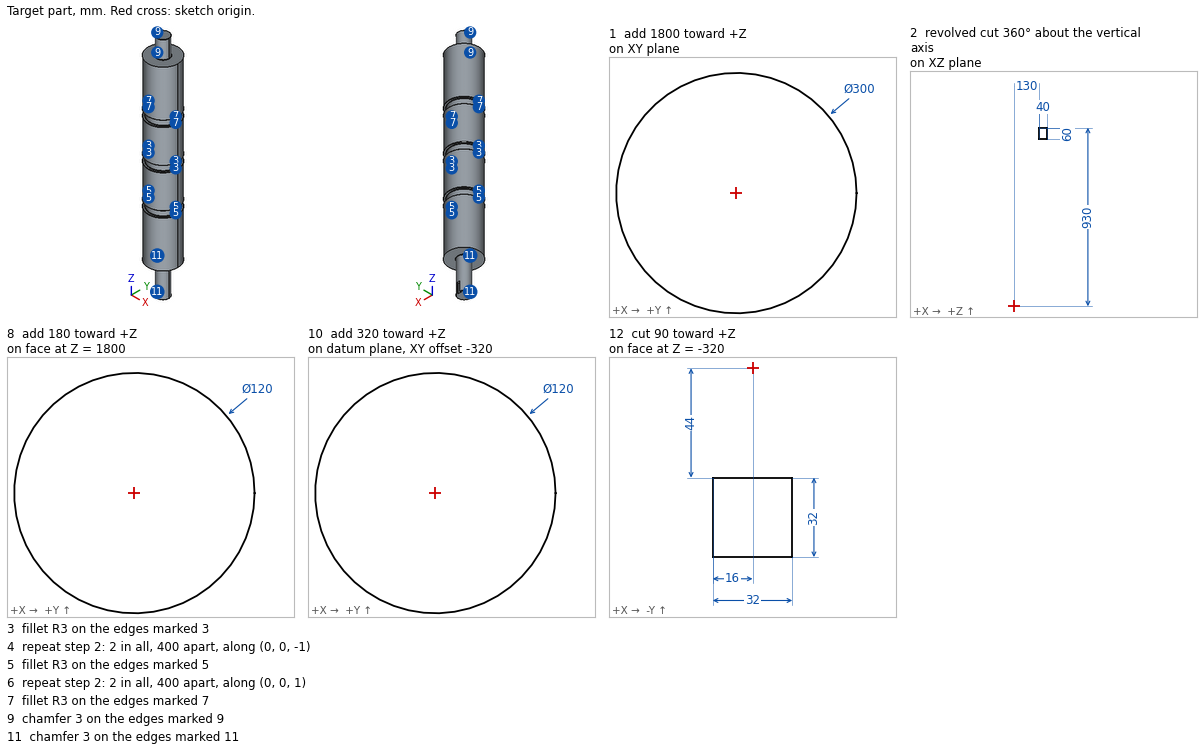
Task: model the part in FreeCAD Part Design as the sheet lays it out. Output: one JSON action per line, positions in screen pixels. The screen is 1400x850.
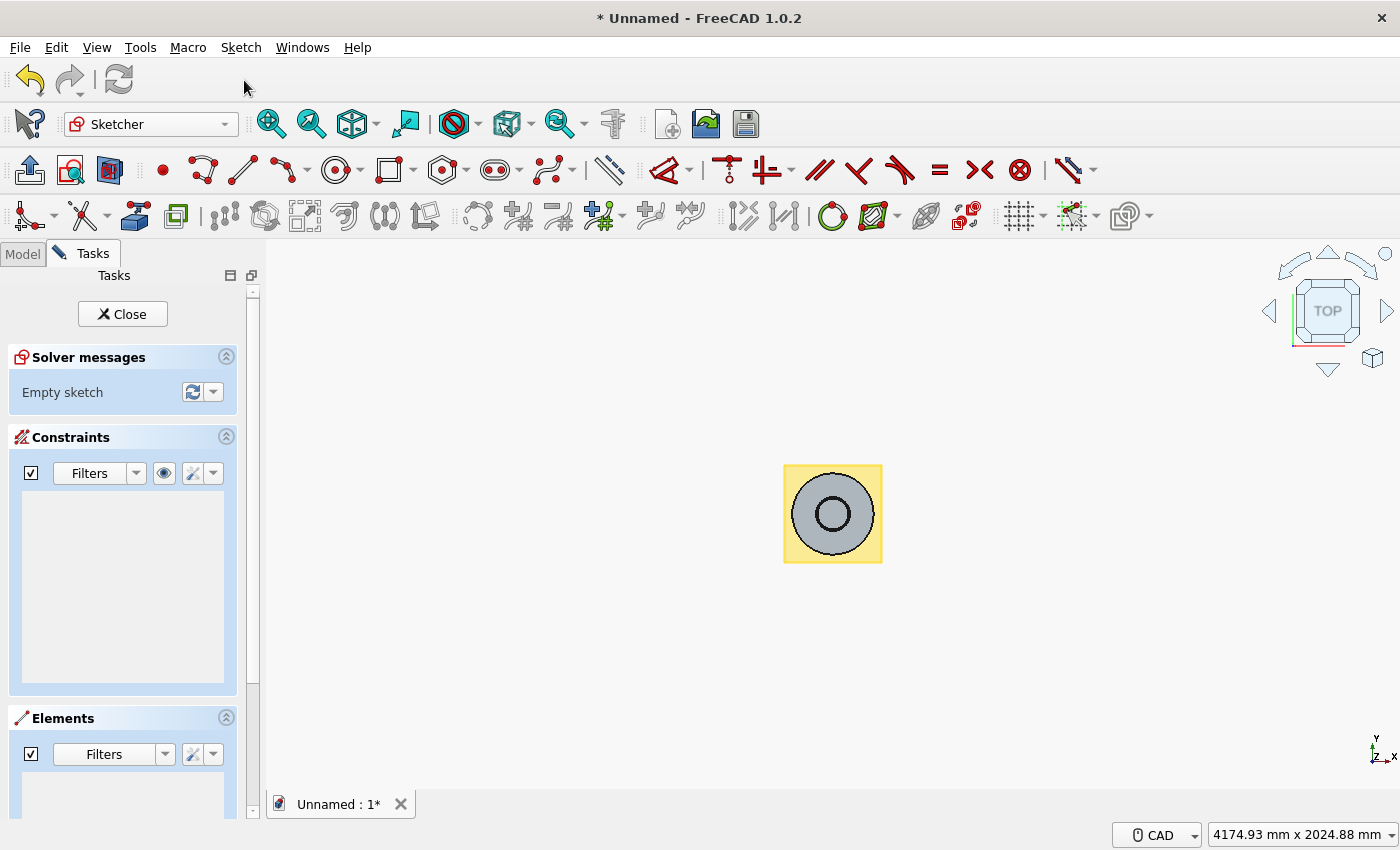
{"action": "left_click", "coordinate": [110, 170]}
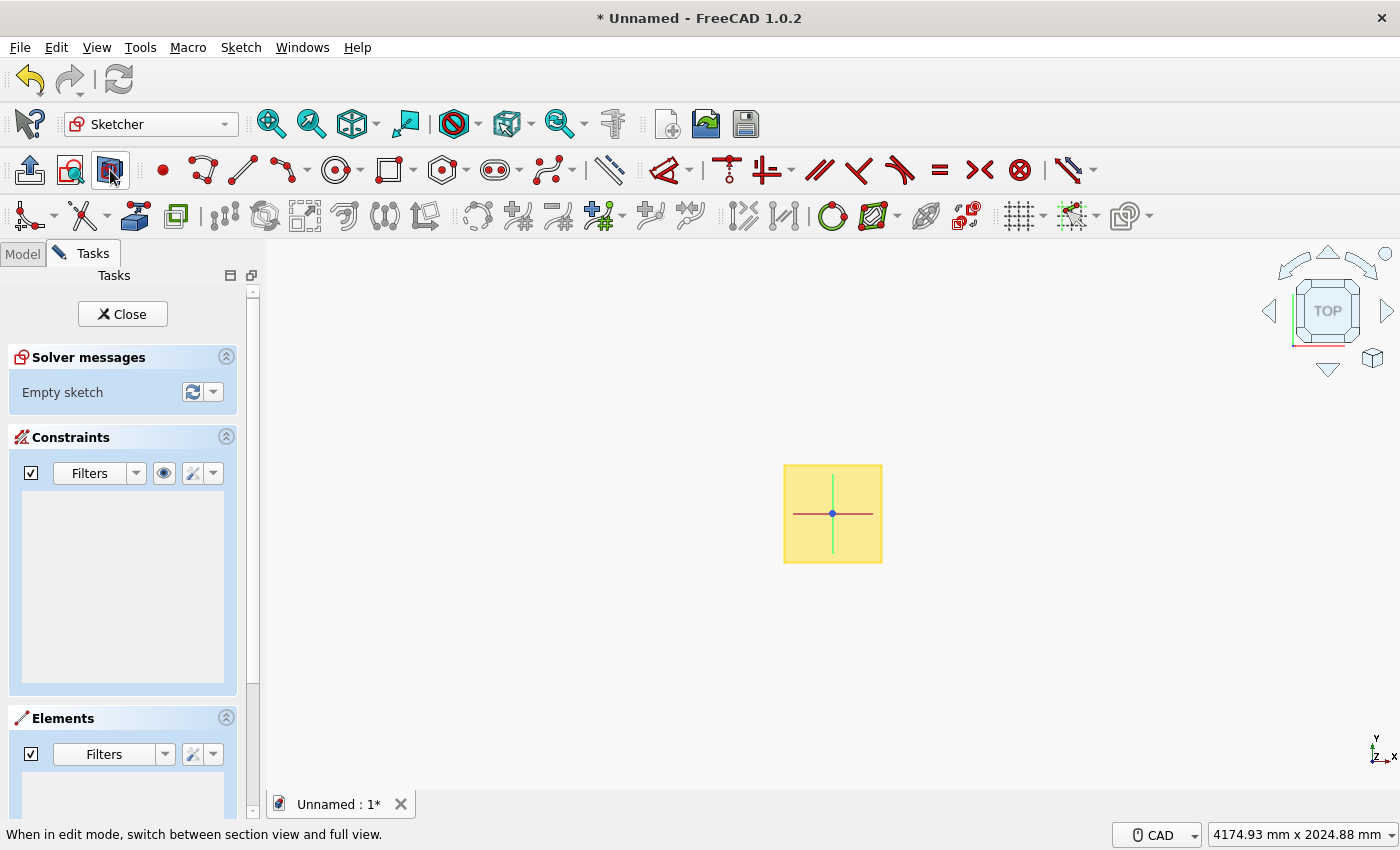
{"action": "scroll", "coordinate": [840, 514], "scroll_direction": "up", "scroll_amount": 12}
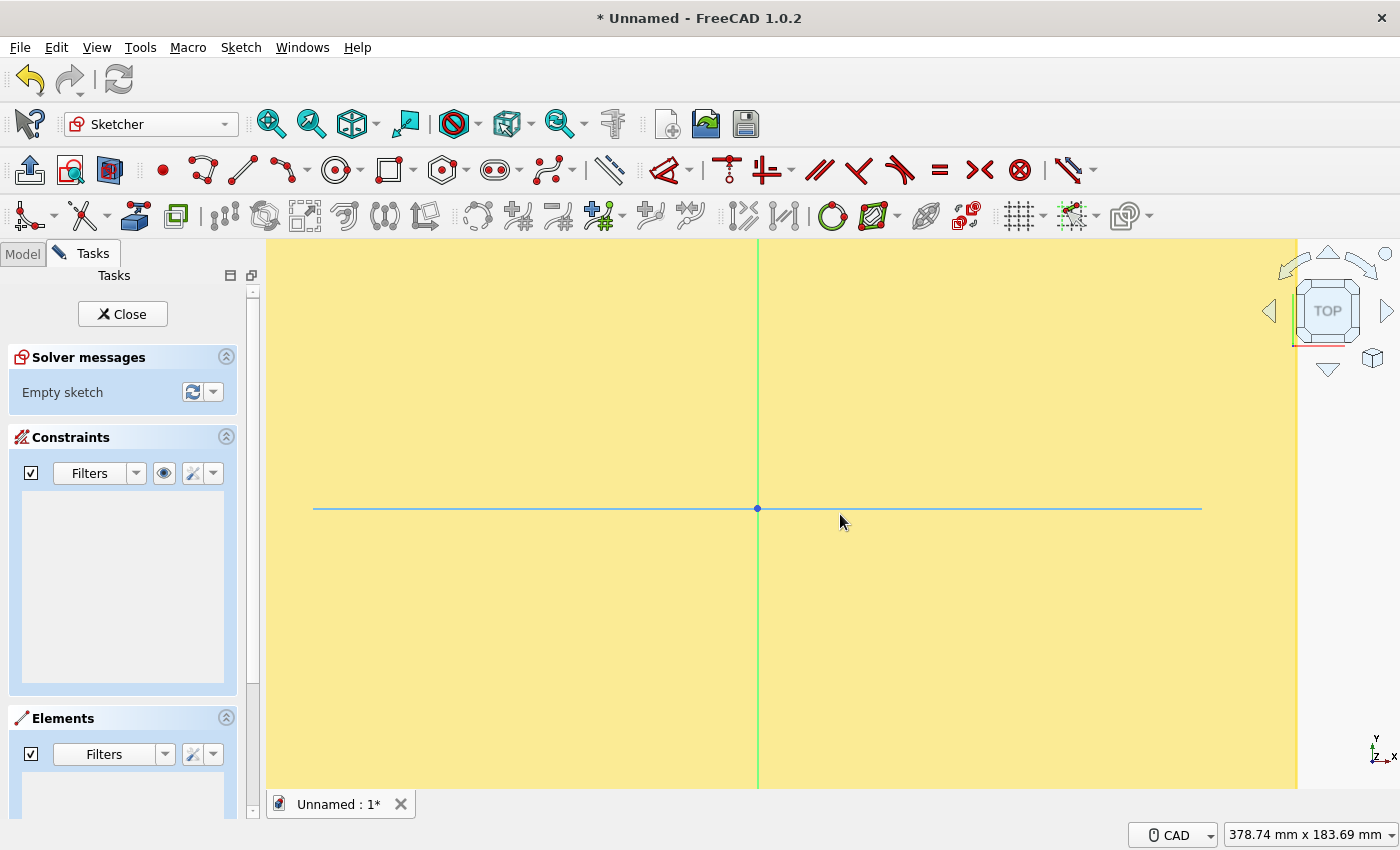
{"action": "left_click", "coordinate": [336, 170]}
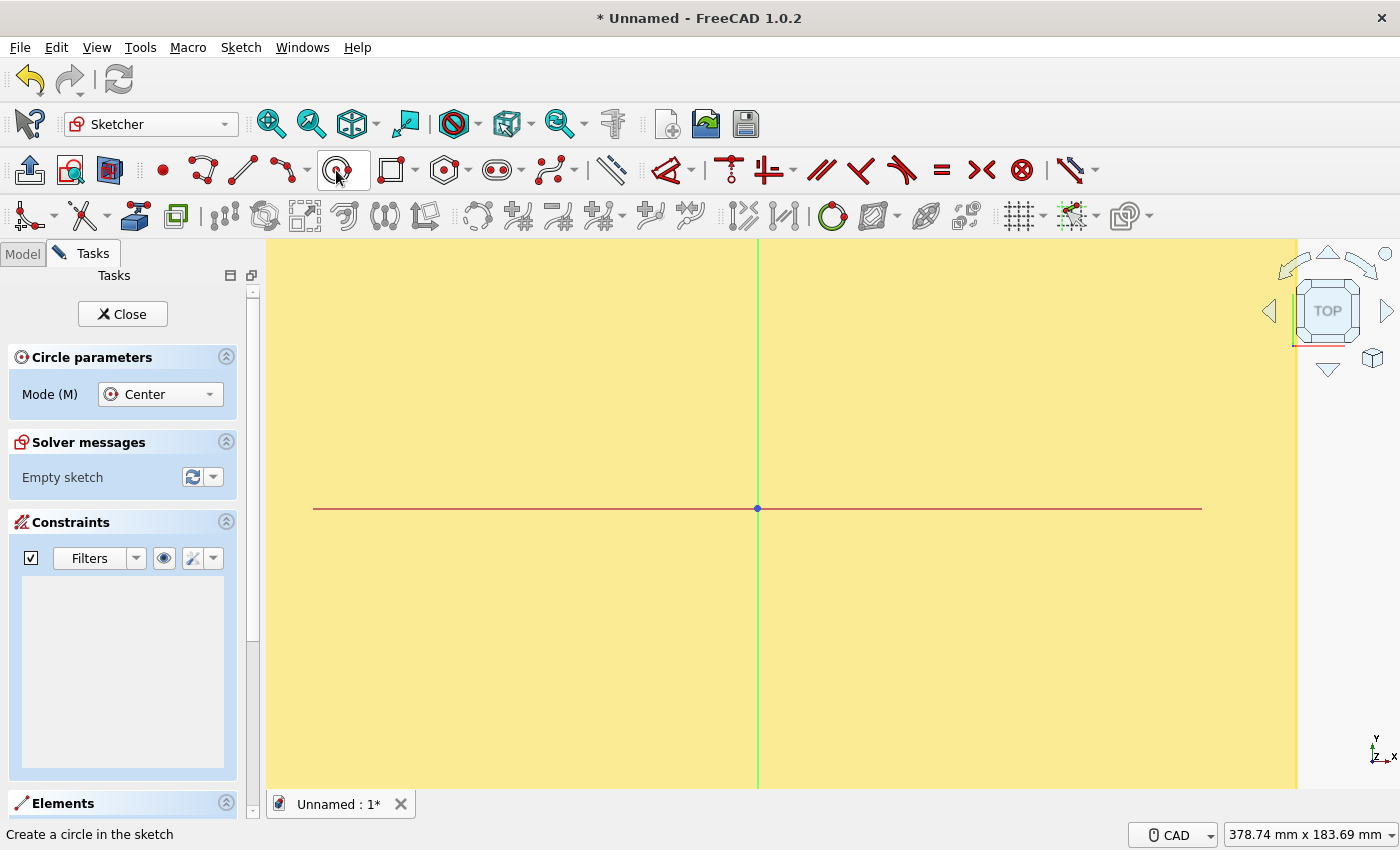
{"action": "left_click", "coordinate": [758, 509]}
{"action": "mouse_move", "coordinate": [885, 382]}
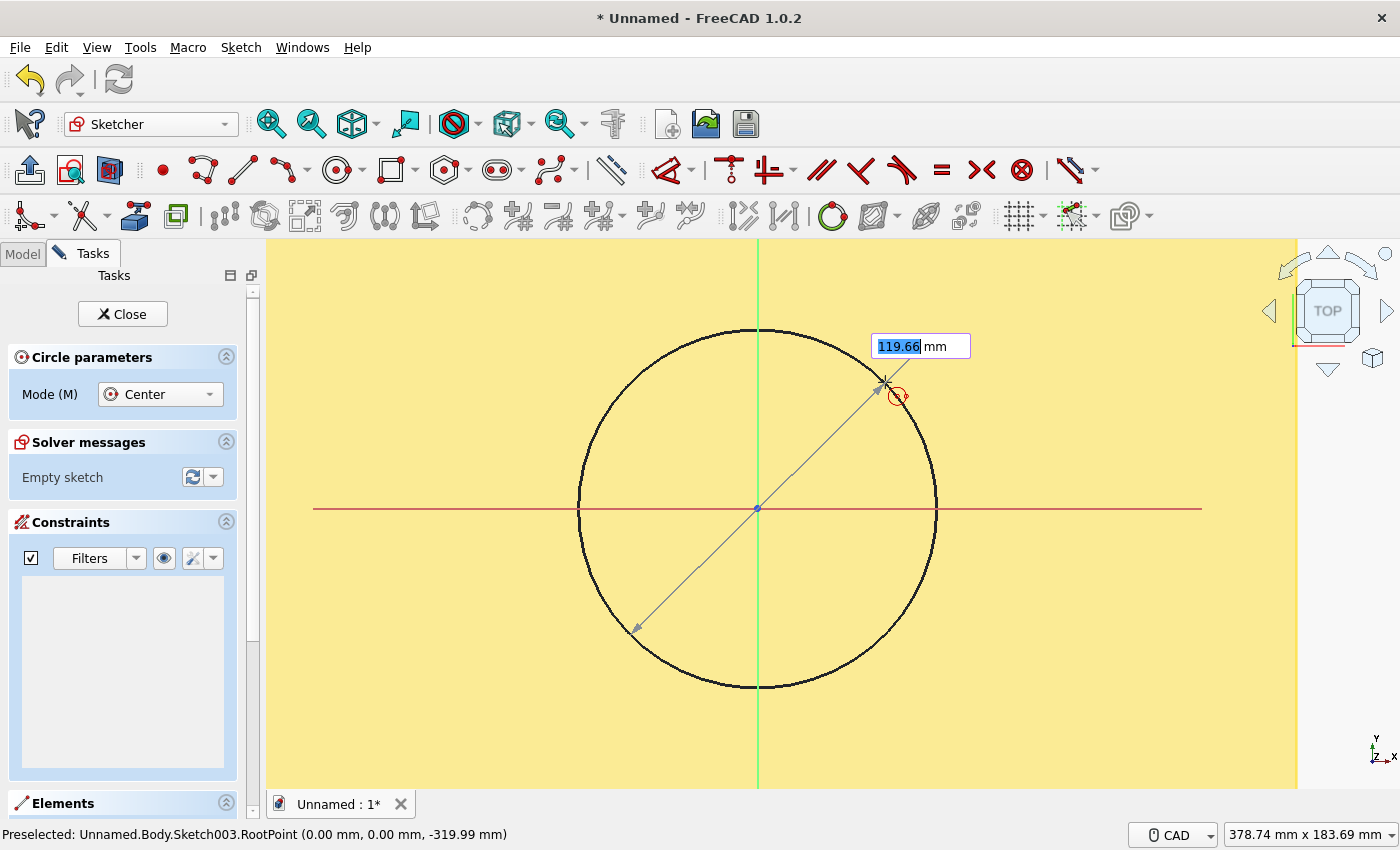
{"action": "type", "text": "120"}
{"action": "key", "text": "Return"}
{"action": "key", "text": "Escape"}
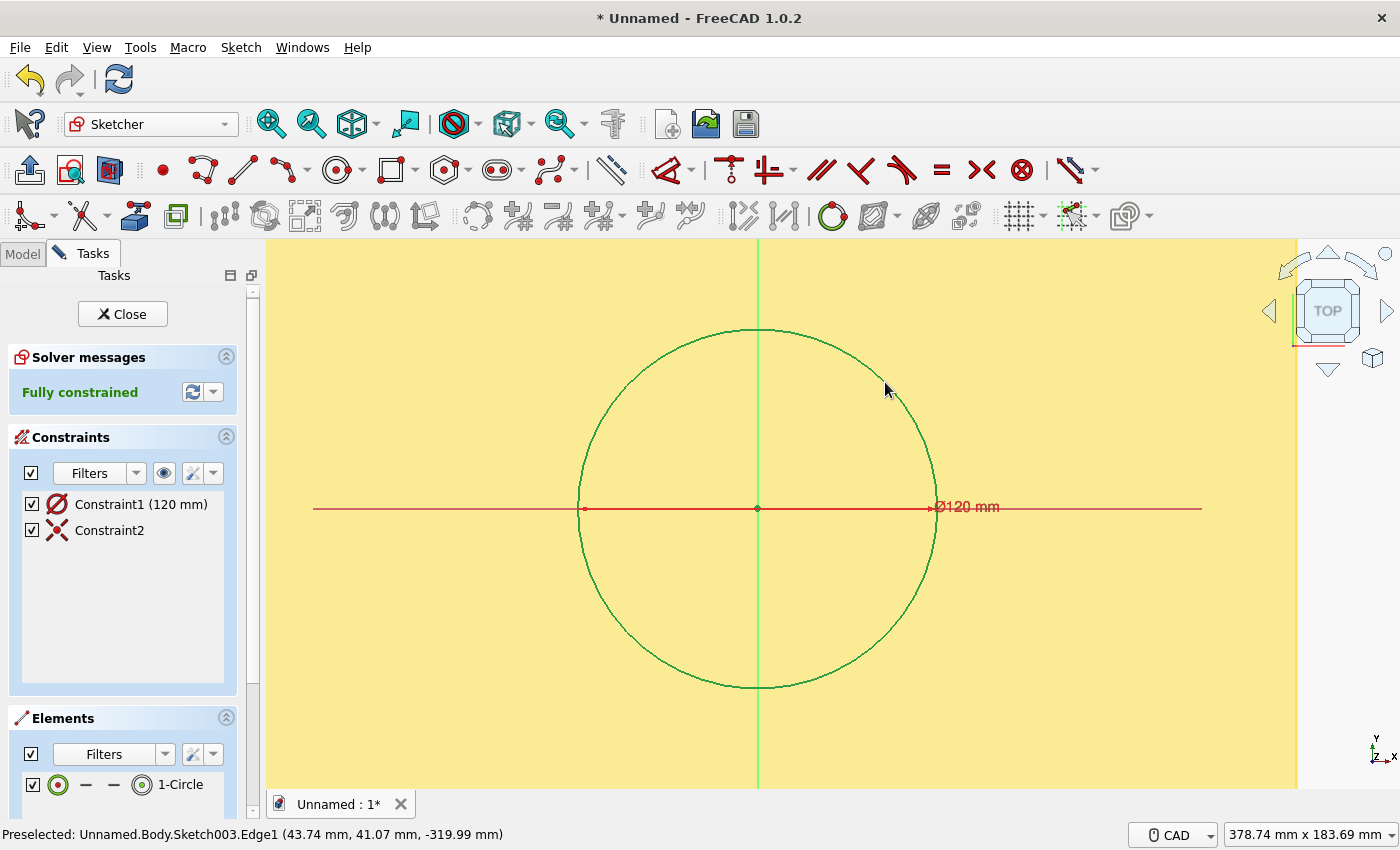
{"action": "left_click", "coordinate": [123, 314]}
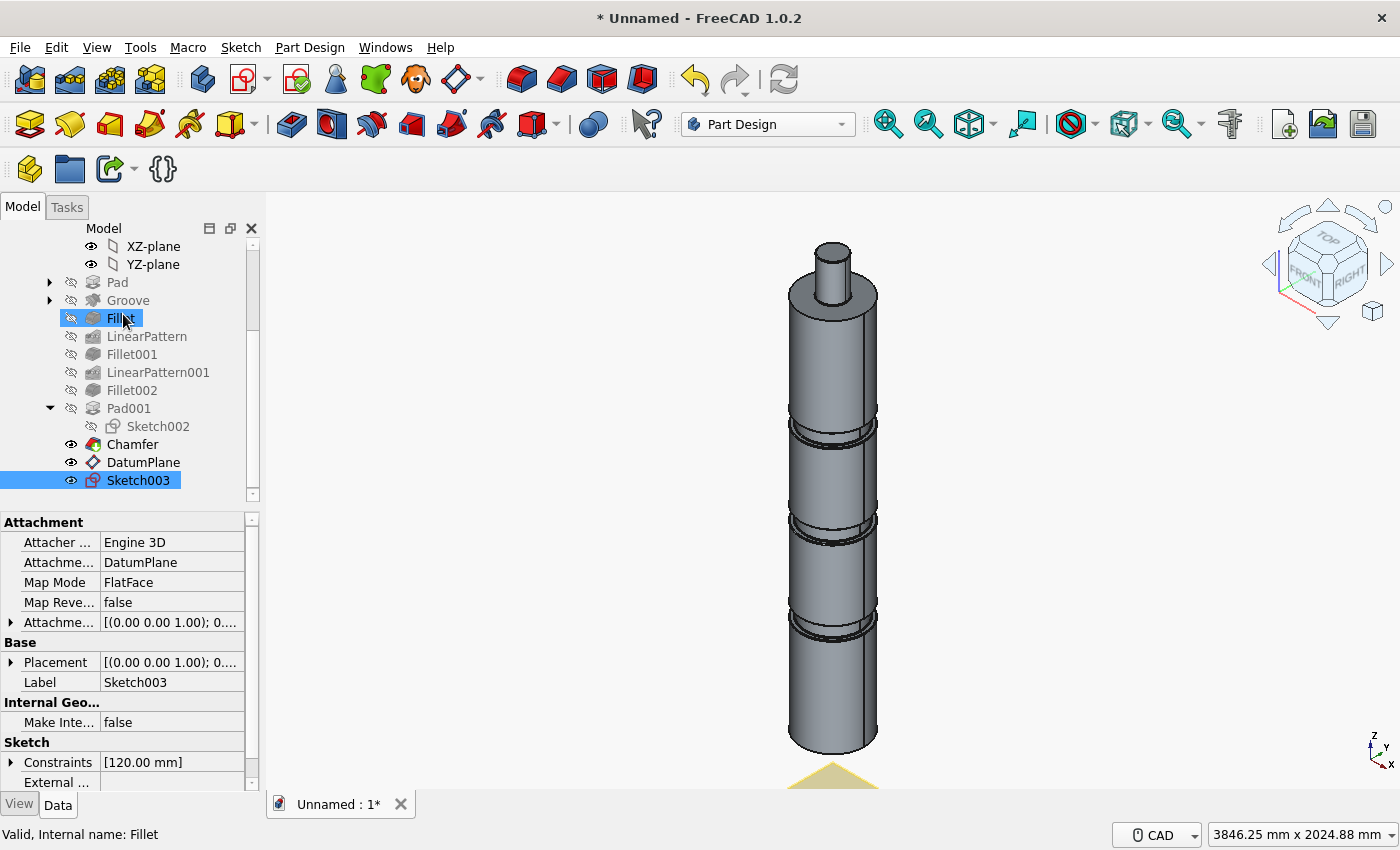
{"action": "left_click", "coordinate": [30, 124]}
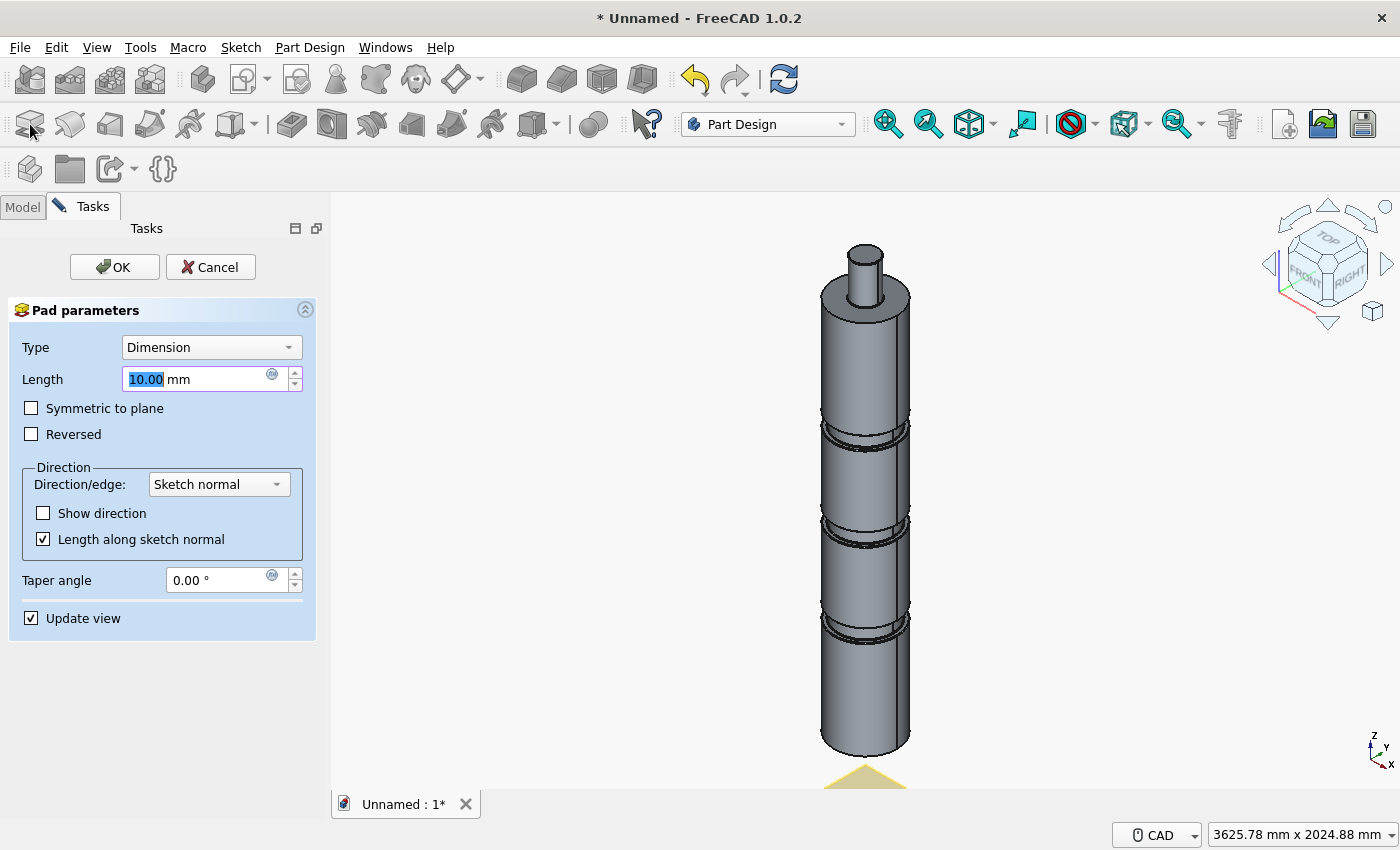
{"action": "type", "text": "320"}
{"action": "key", "text": "Tab"}